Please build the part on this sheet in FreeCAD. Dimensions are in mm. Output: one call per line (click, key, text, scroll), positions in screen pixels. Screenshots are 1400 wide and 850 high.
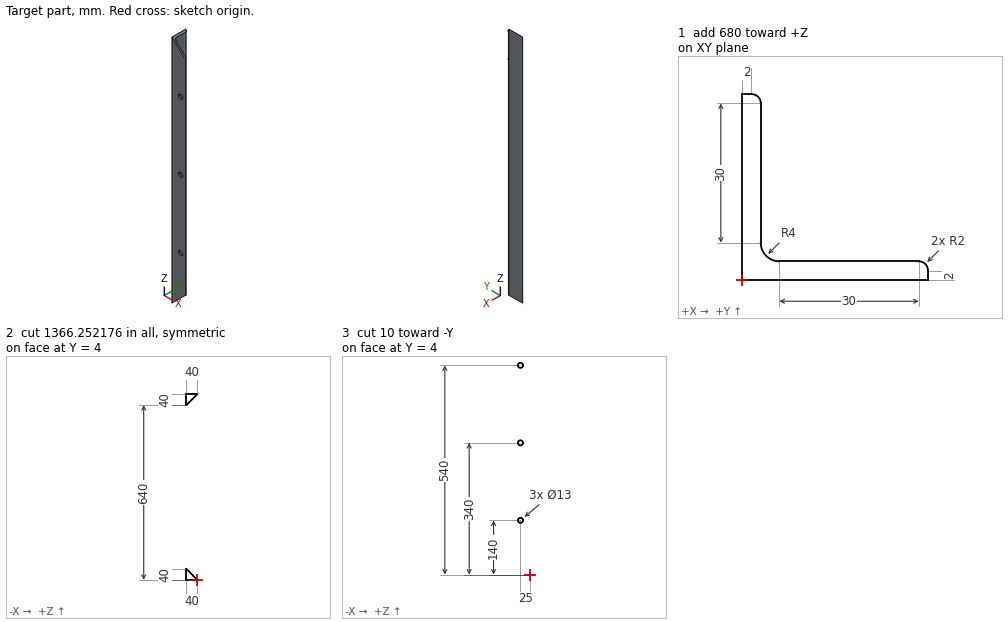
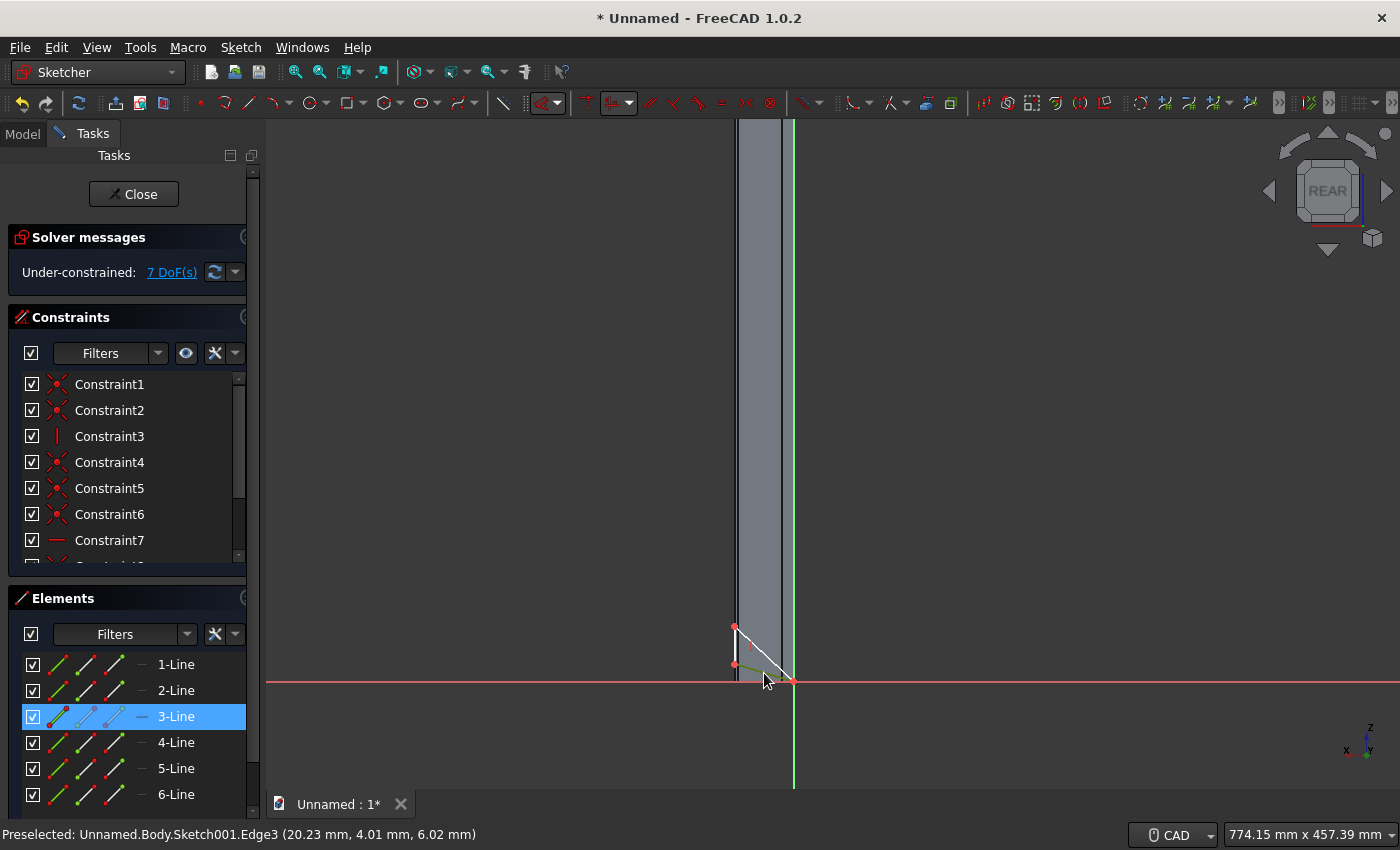
click(632, 104)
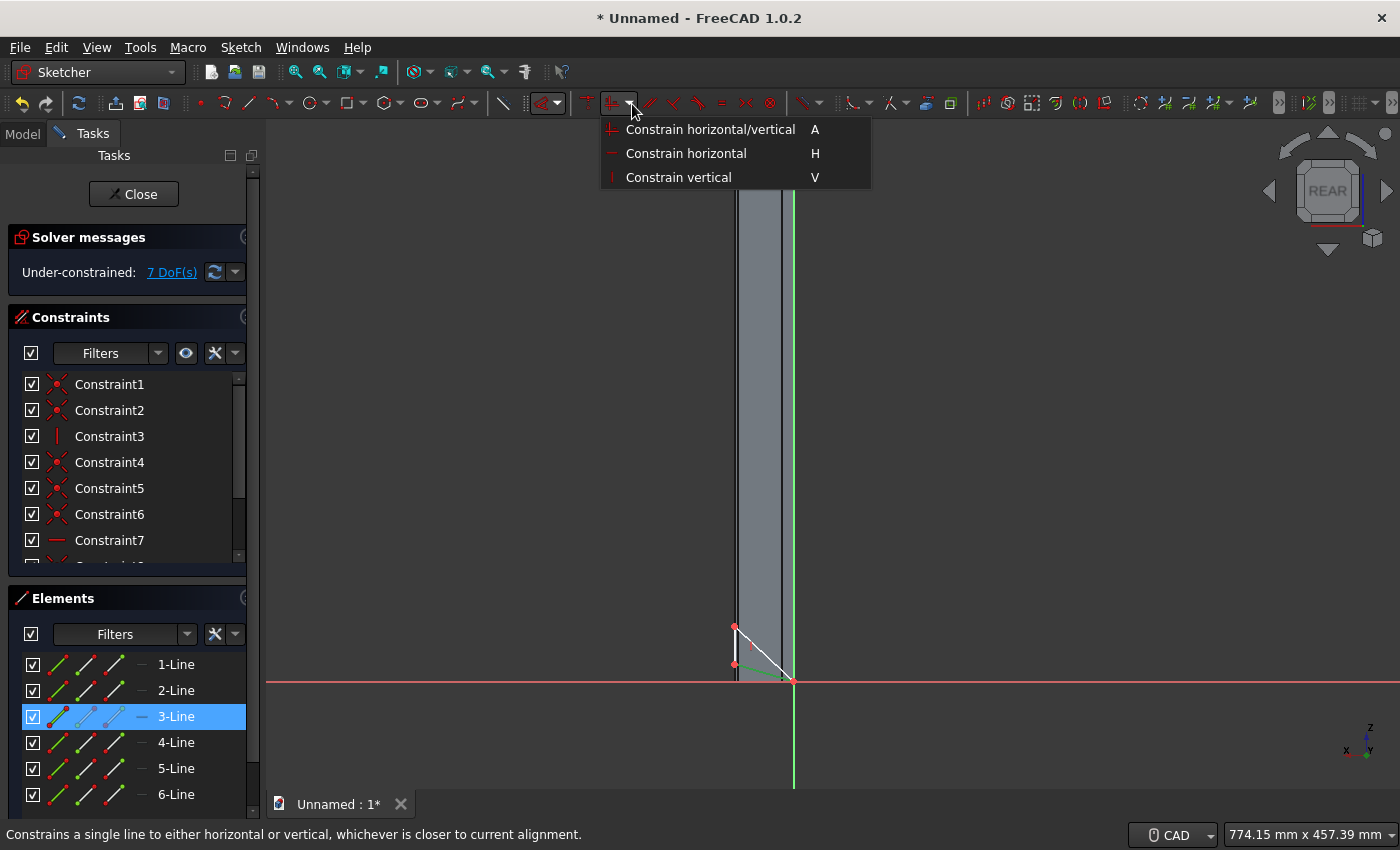
click(736, 153)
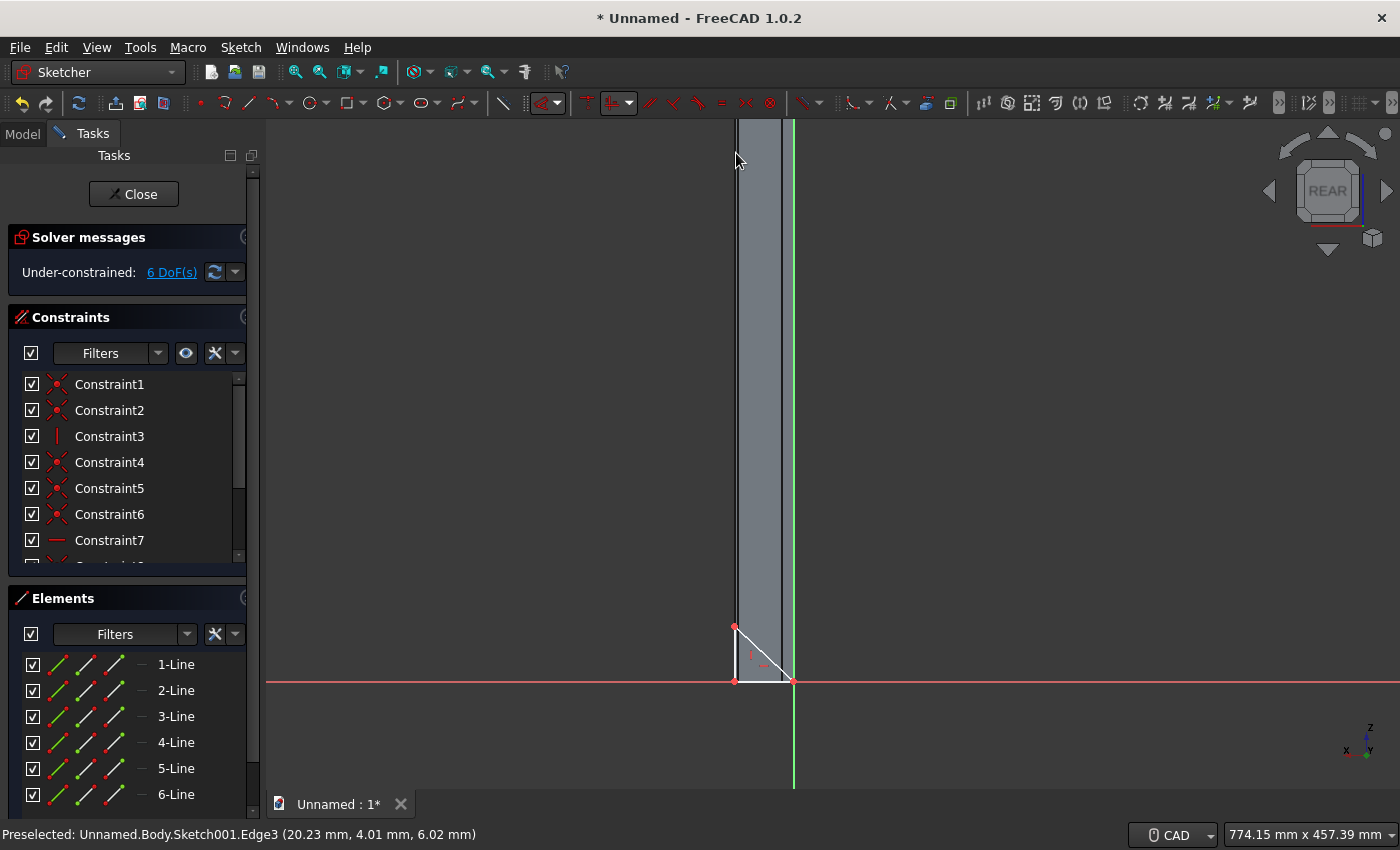
scroll(764, 675, down, 4)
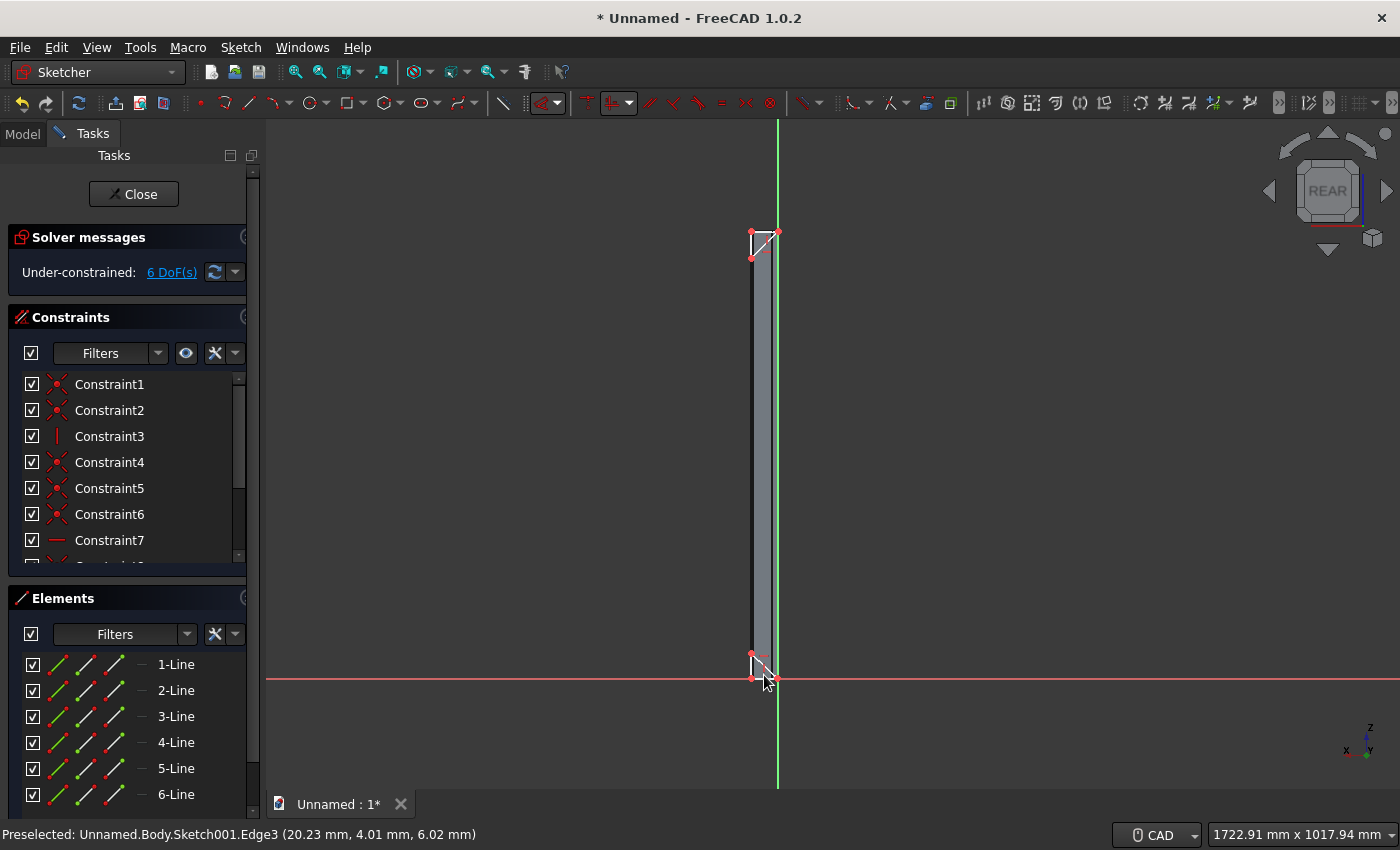
click(778, 232)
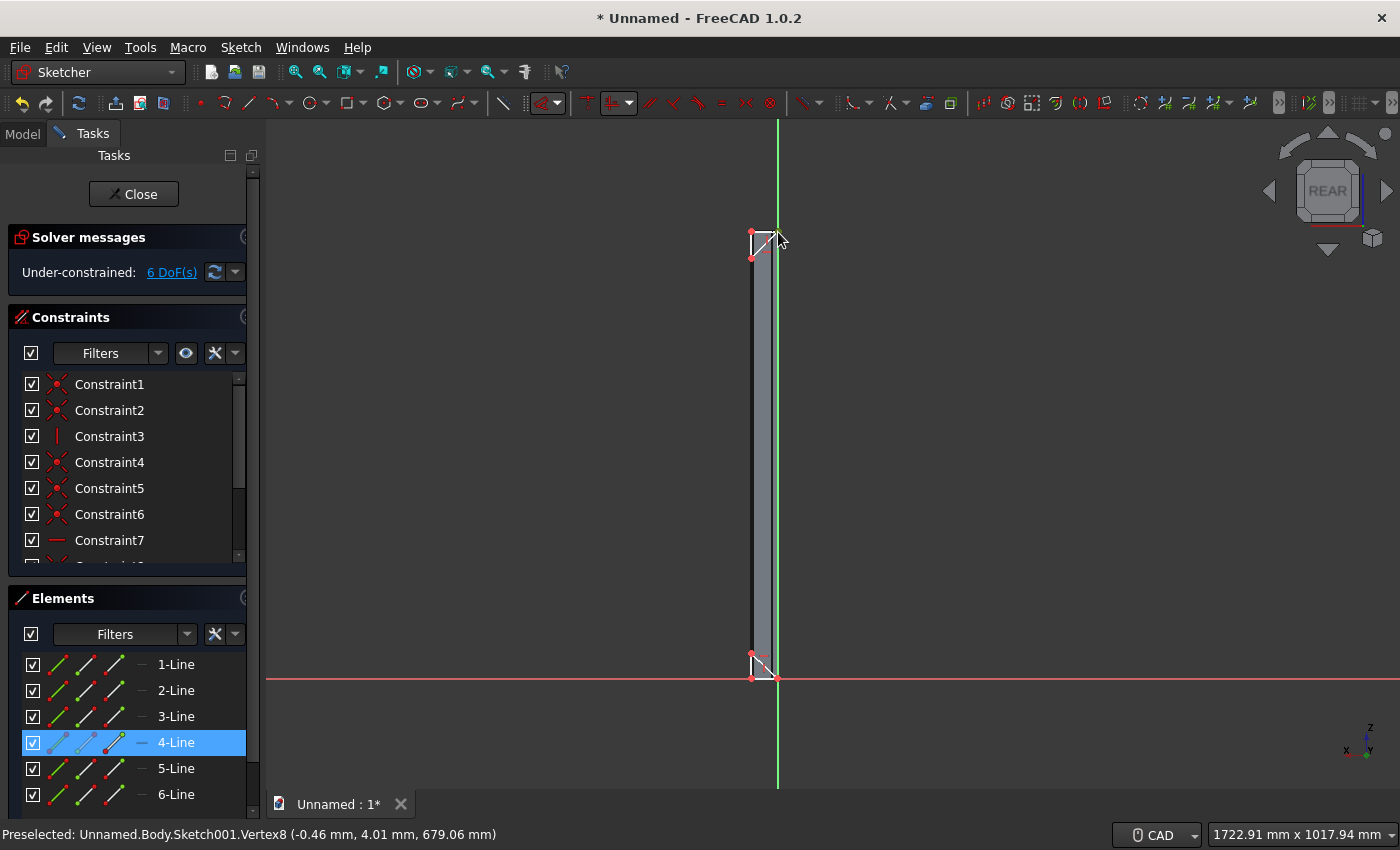
click(778, 717)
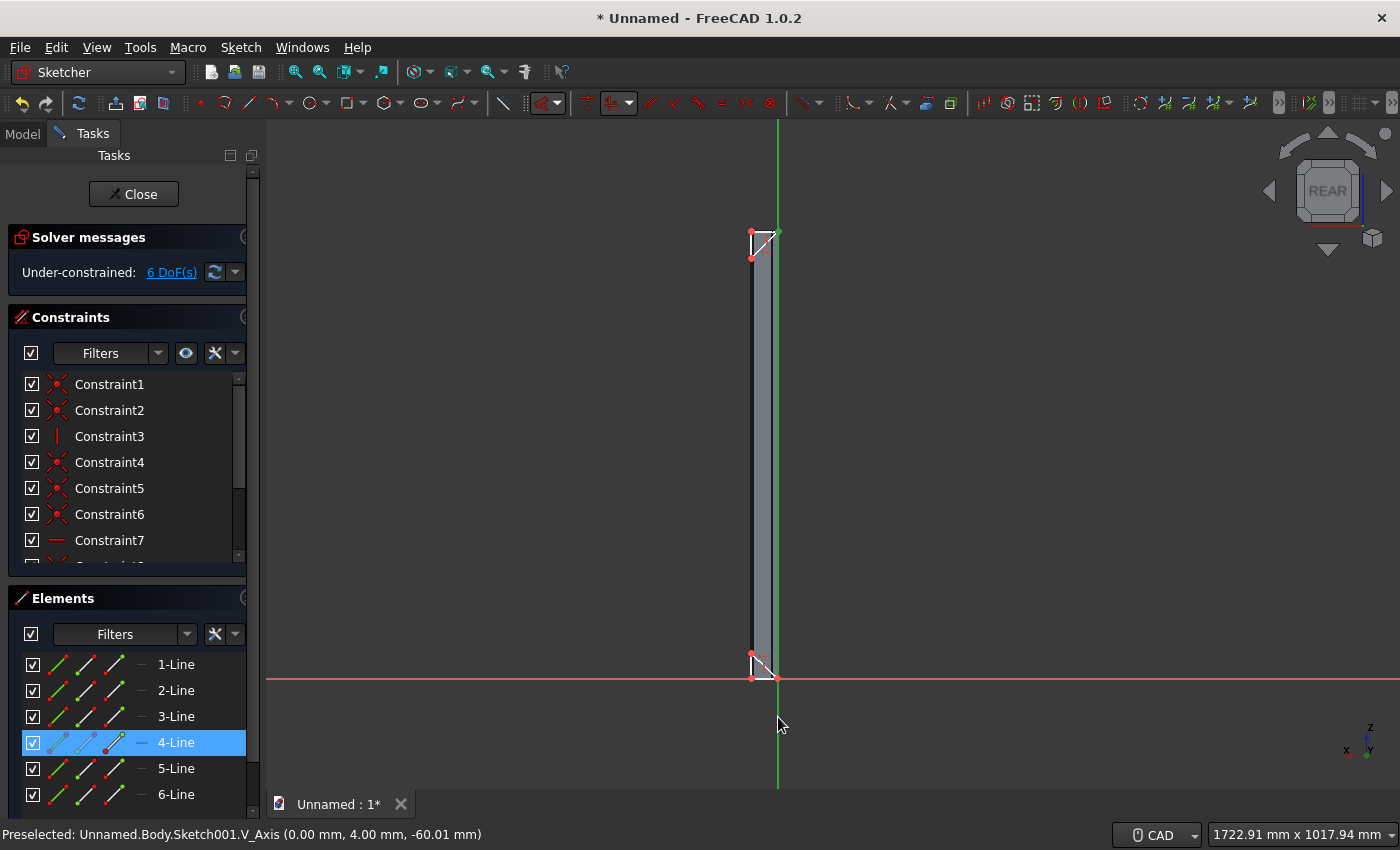
click(588, 104)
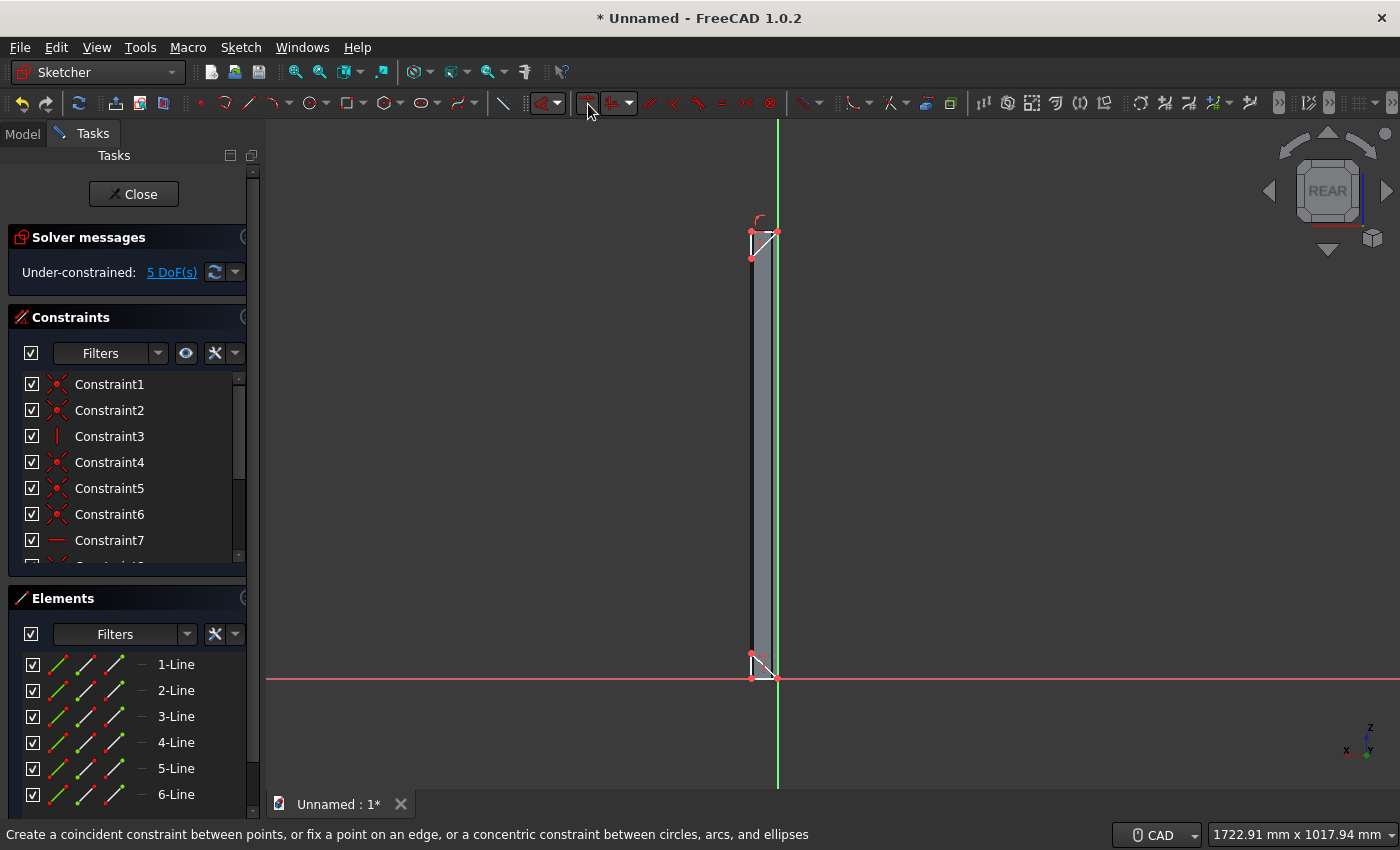
scroll(751, 669, up, 3)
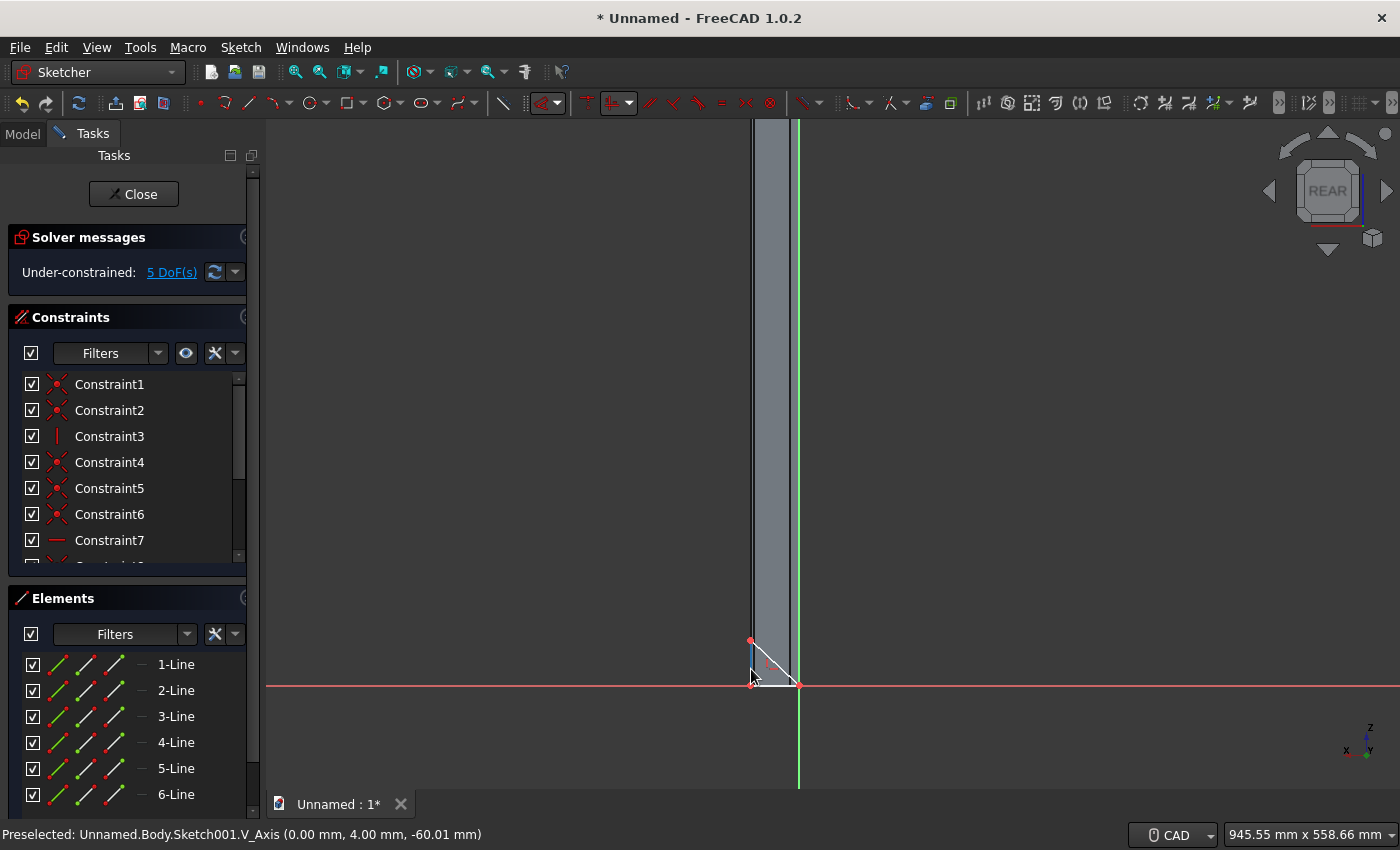
click(751, 667)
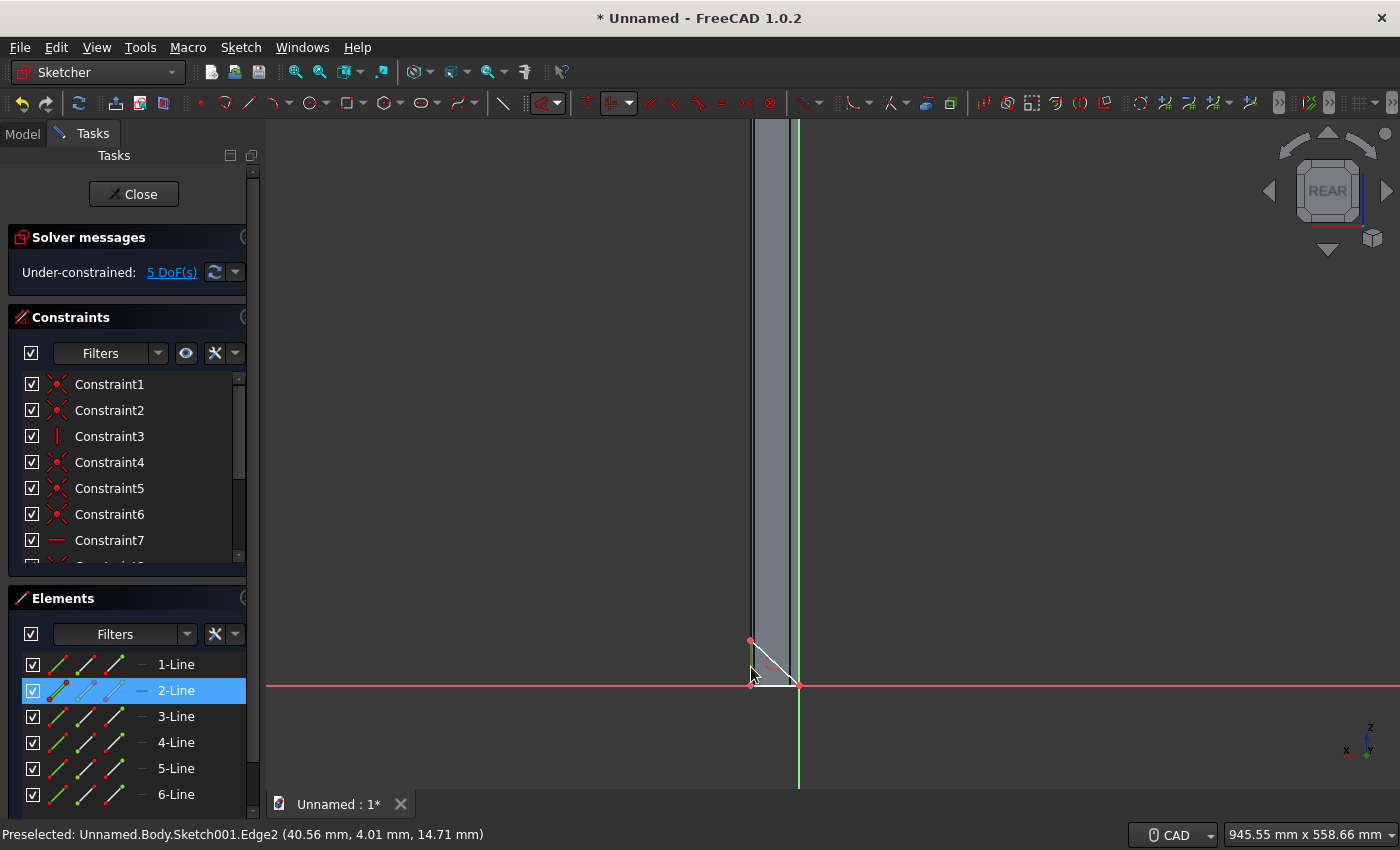
click(560, 104)